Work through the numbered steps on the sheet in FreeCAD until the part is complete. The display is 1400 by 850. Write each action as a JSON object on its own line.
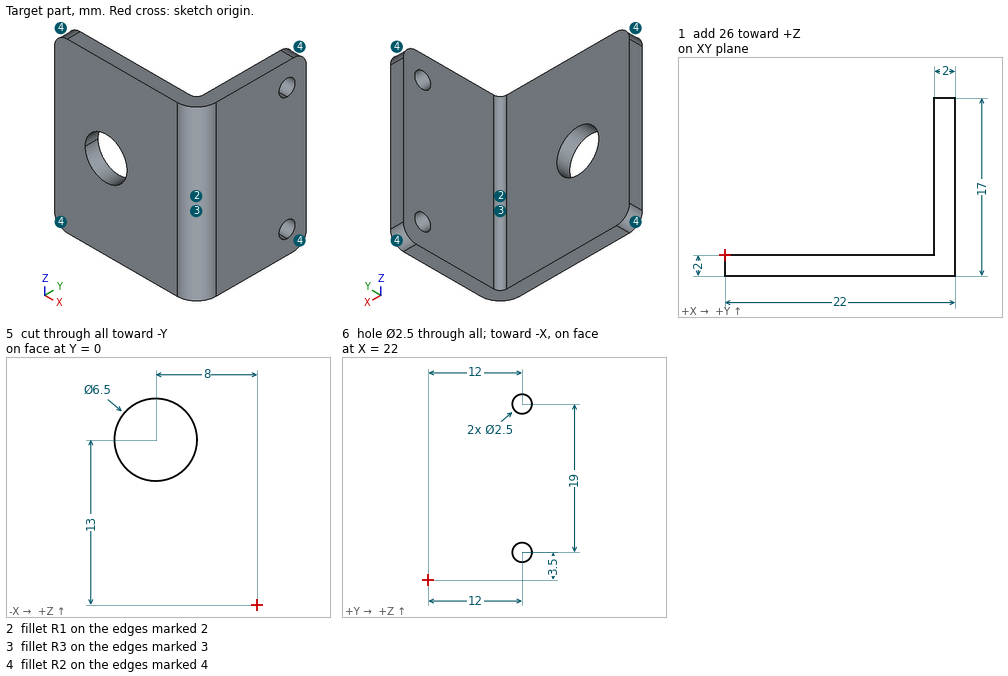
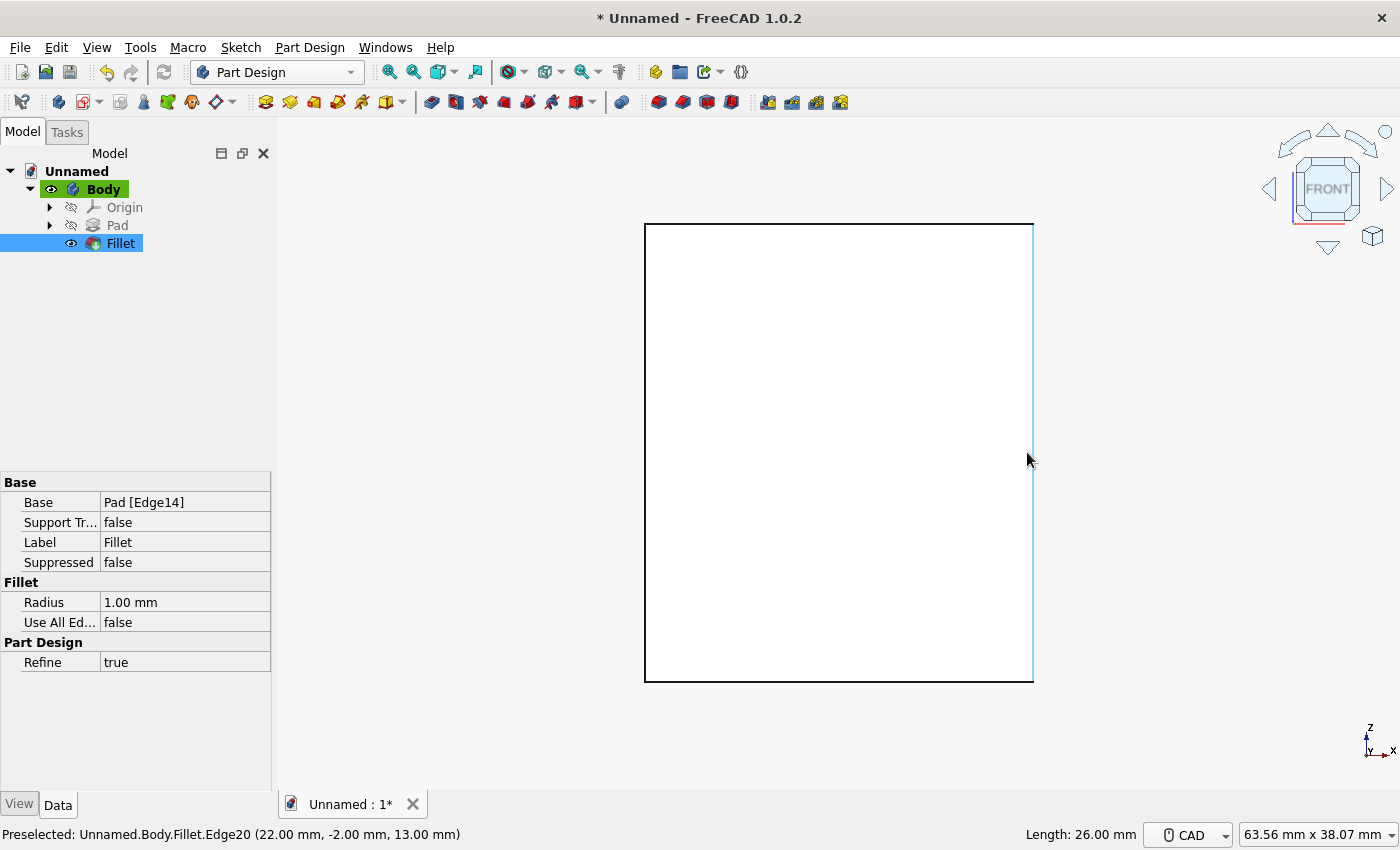
{"action": "left_click", "coordinate": [660, 102]}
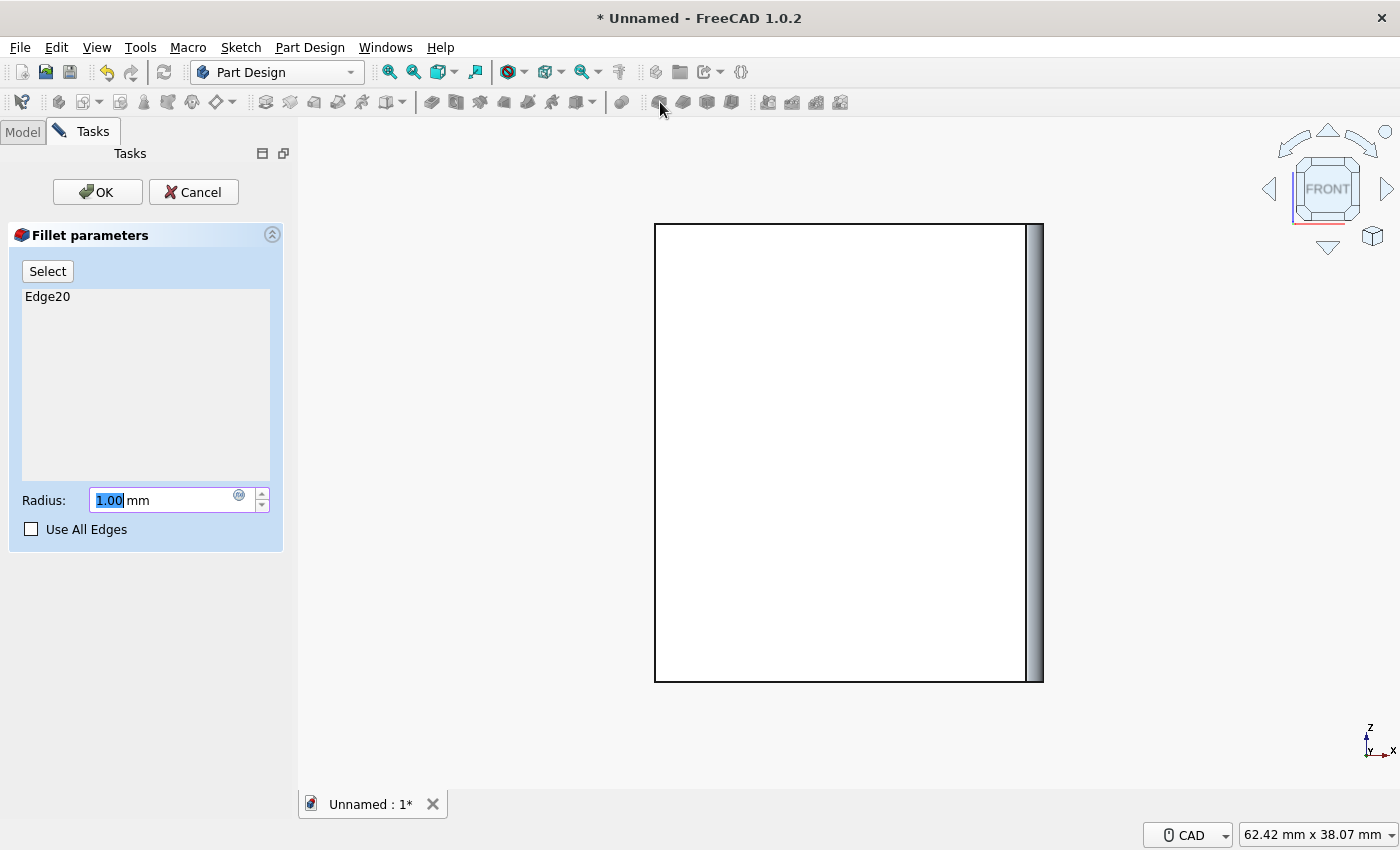
{"action": "type", "text": "3"}
{"action": "key", "text": "Tab"}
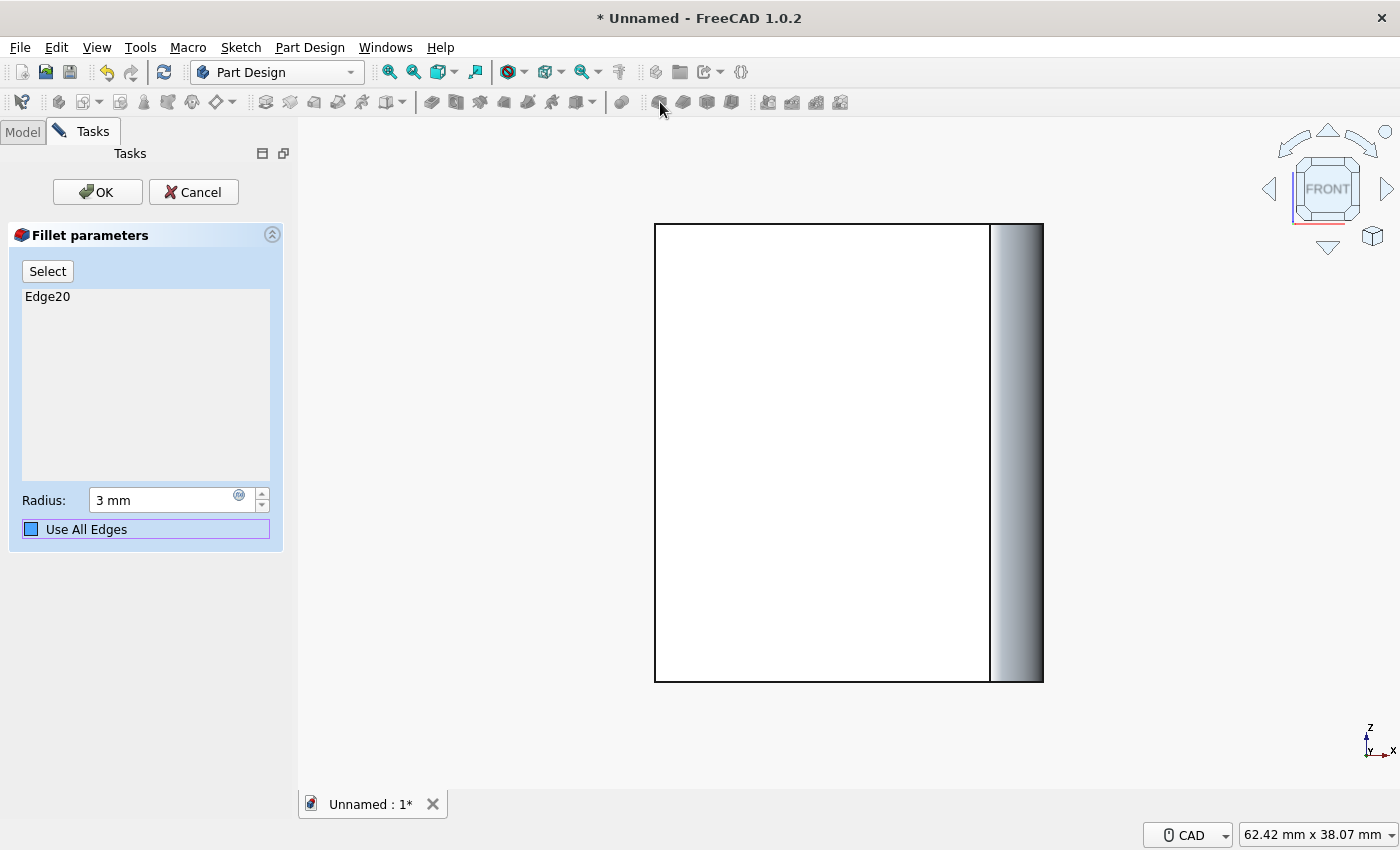
{"action": "left_click", "coordinate": [98, 192]}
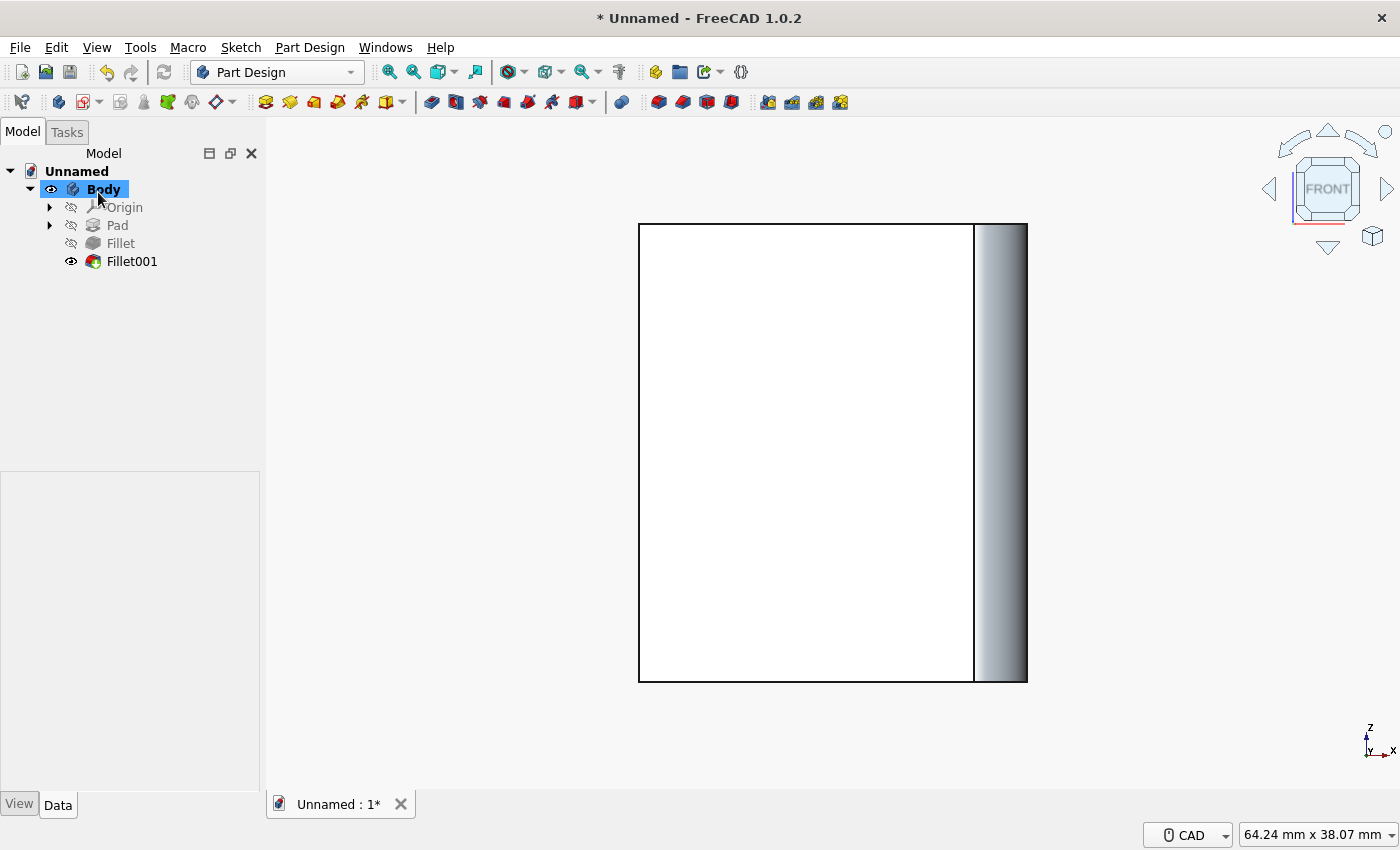
{"action": "key", "text": "0"}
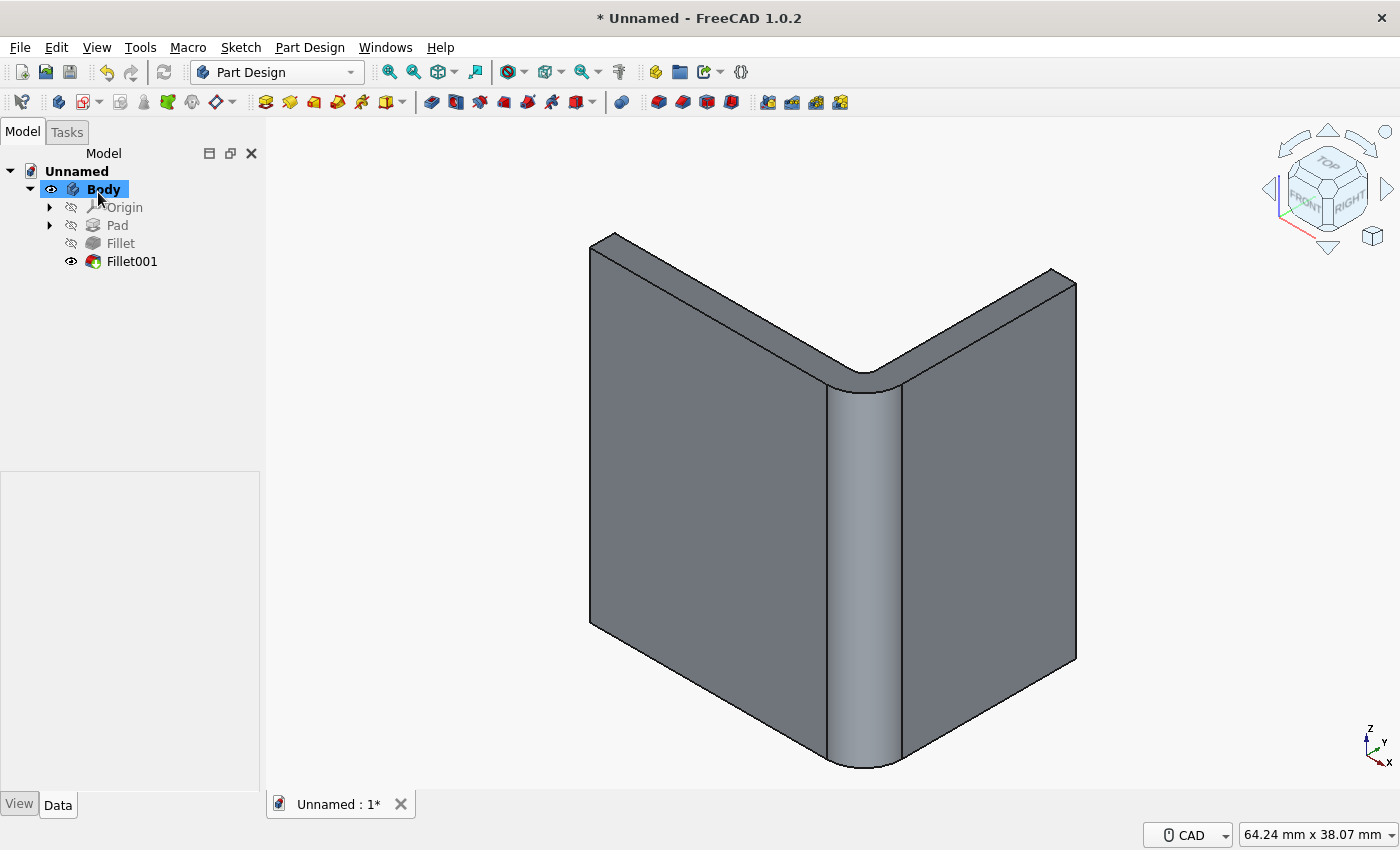
{"action": "key", "text": "2"}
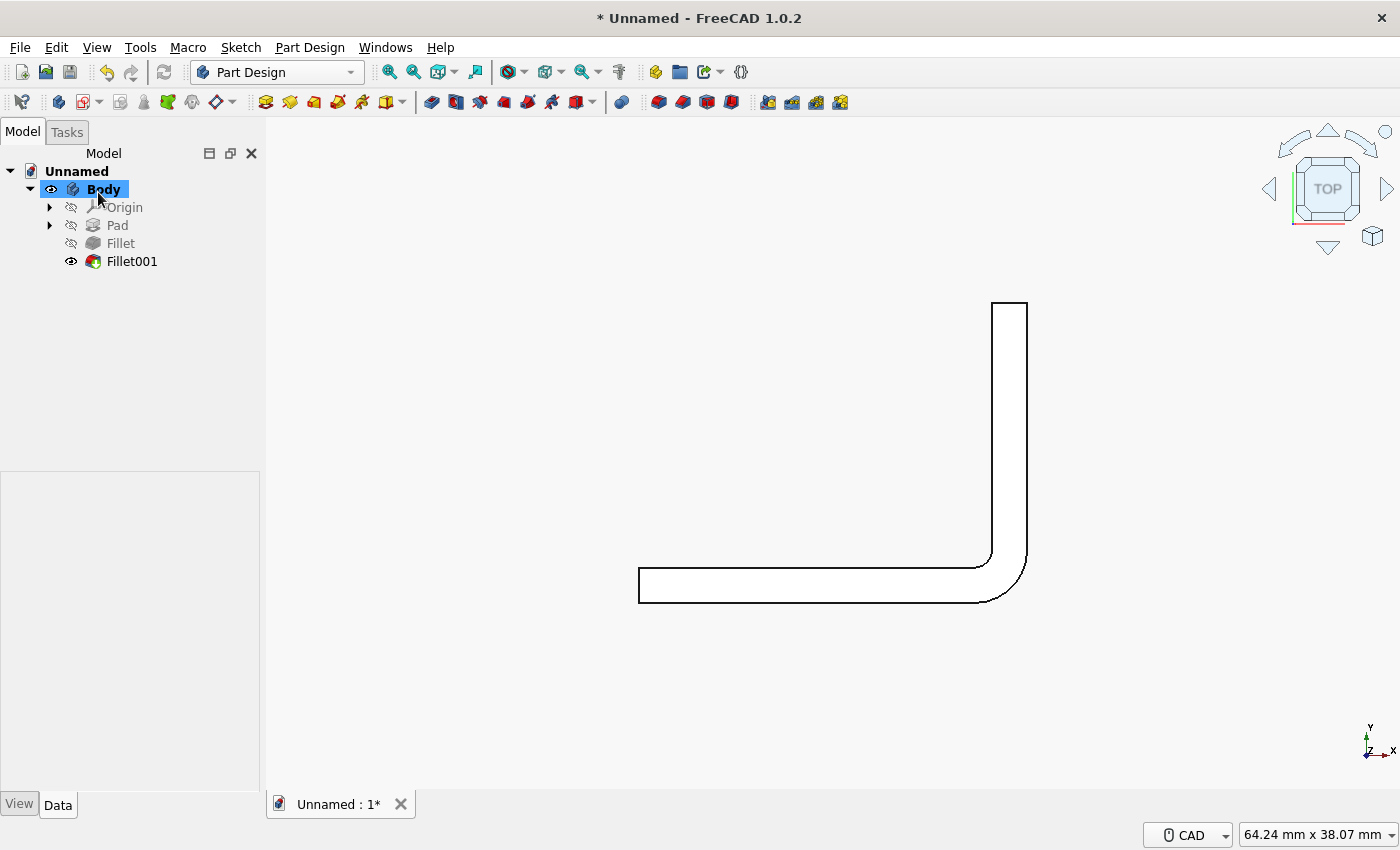
{"action": "left_click", "coordinate": [390, 72]}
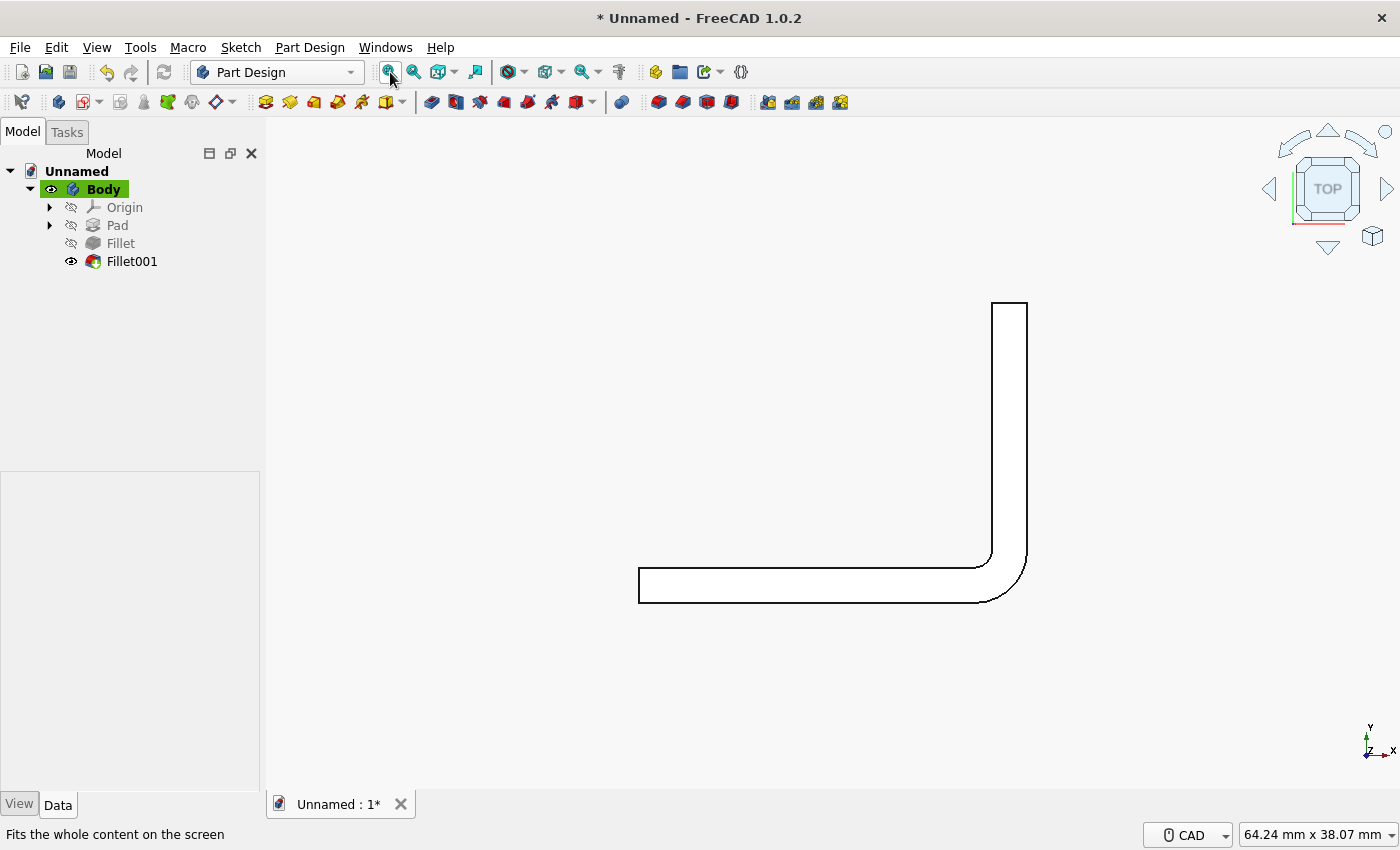
{"action": "left_click", "coordinate": [639, 584]}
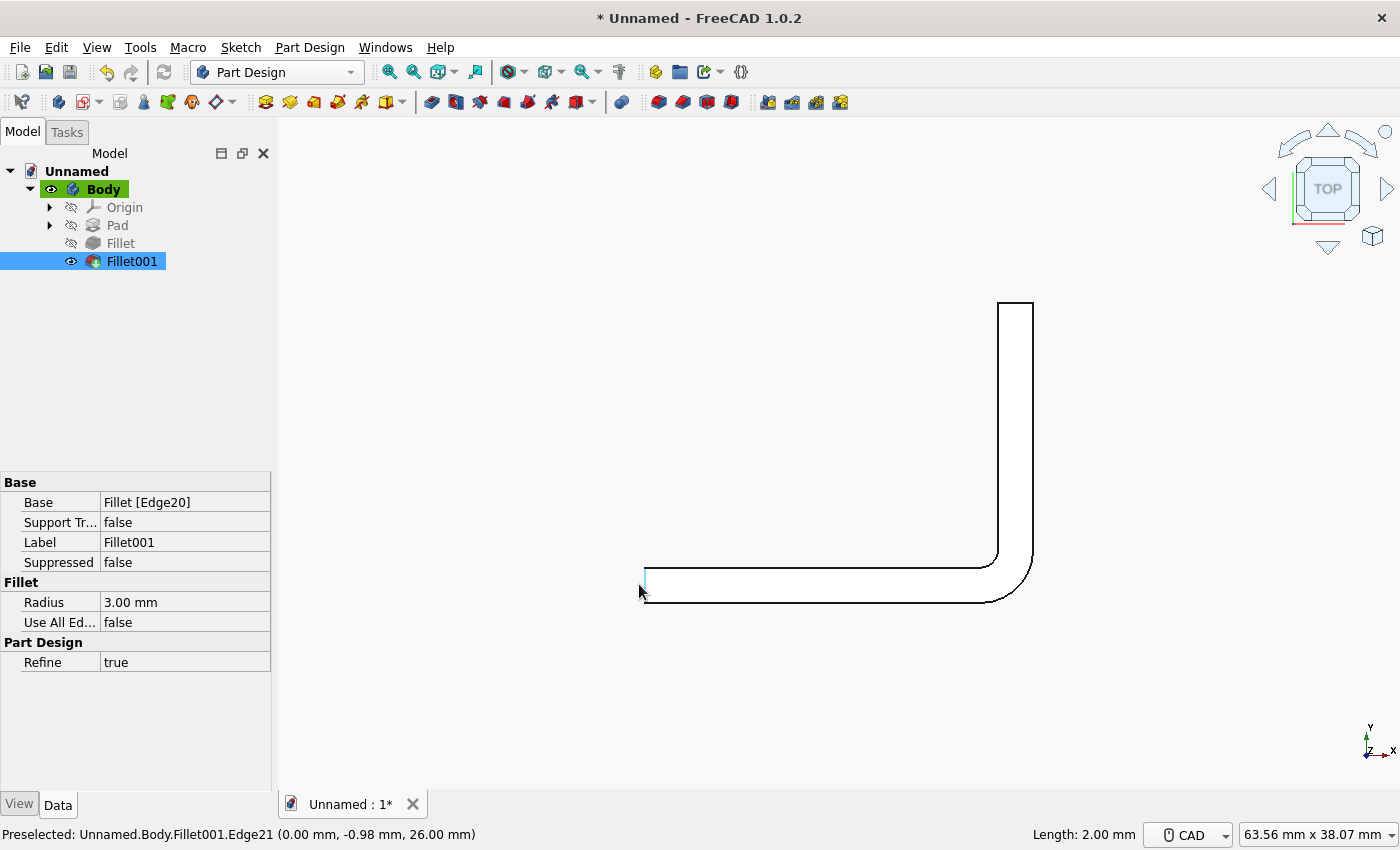
{"action": "left_click", "coordinate": [1016, 302], "text": "ctrl"}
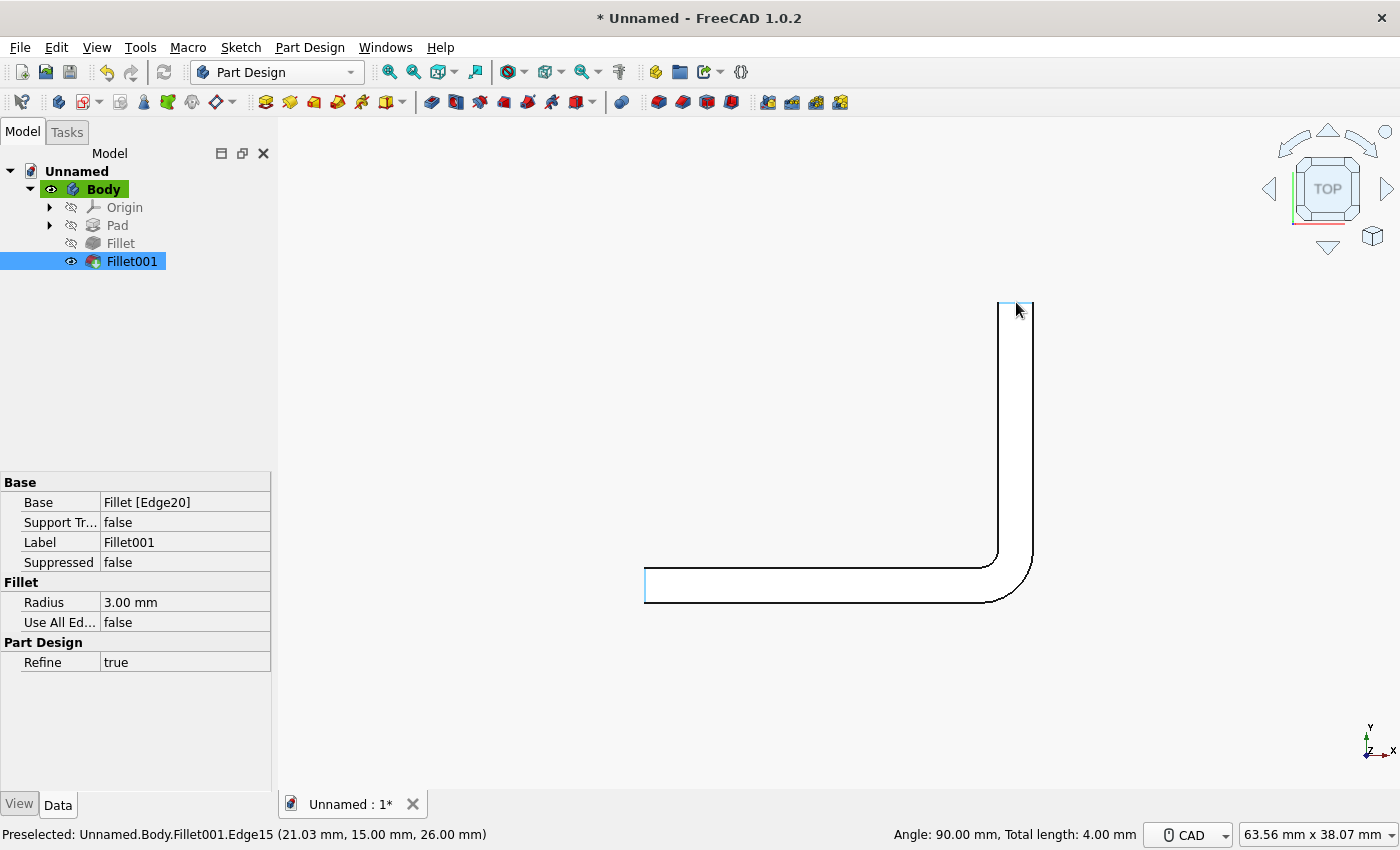
{"action": "key", "text": "1"}